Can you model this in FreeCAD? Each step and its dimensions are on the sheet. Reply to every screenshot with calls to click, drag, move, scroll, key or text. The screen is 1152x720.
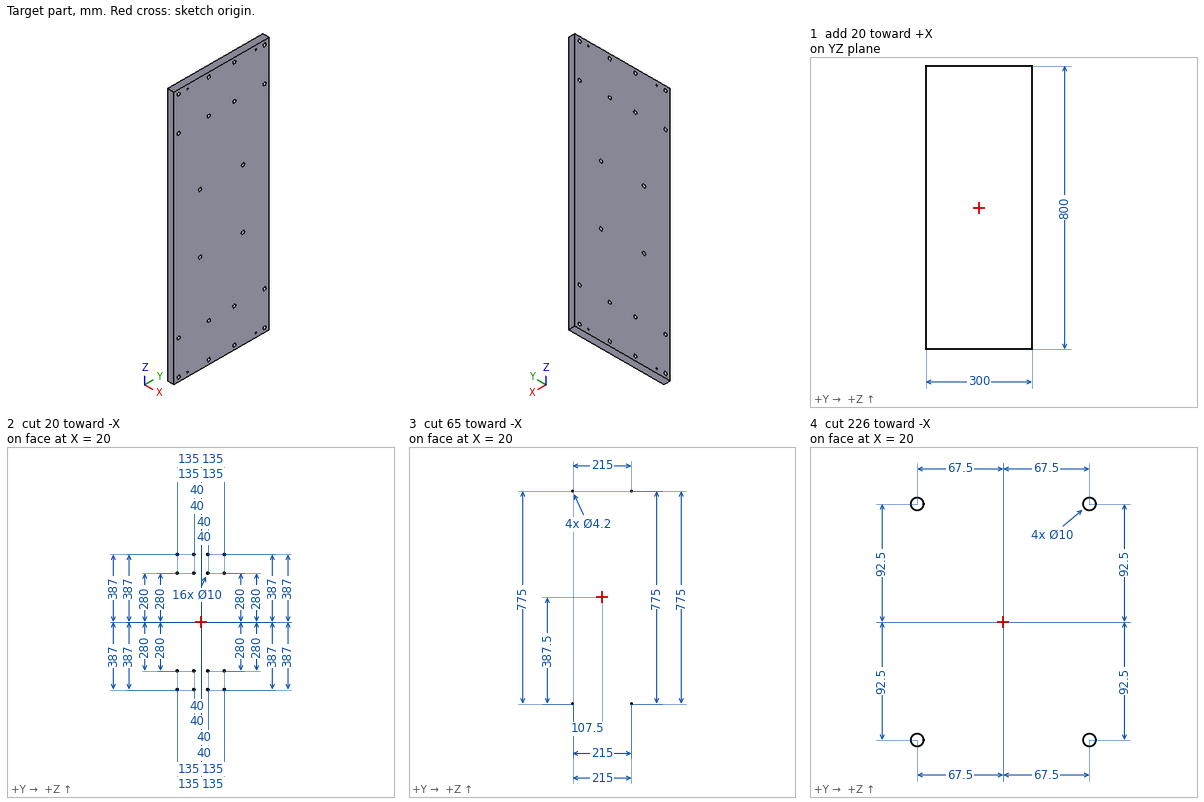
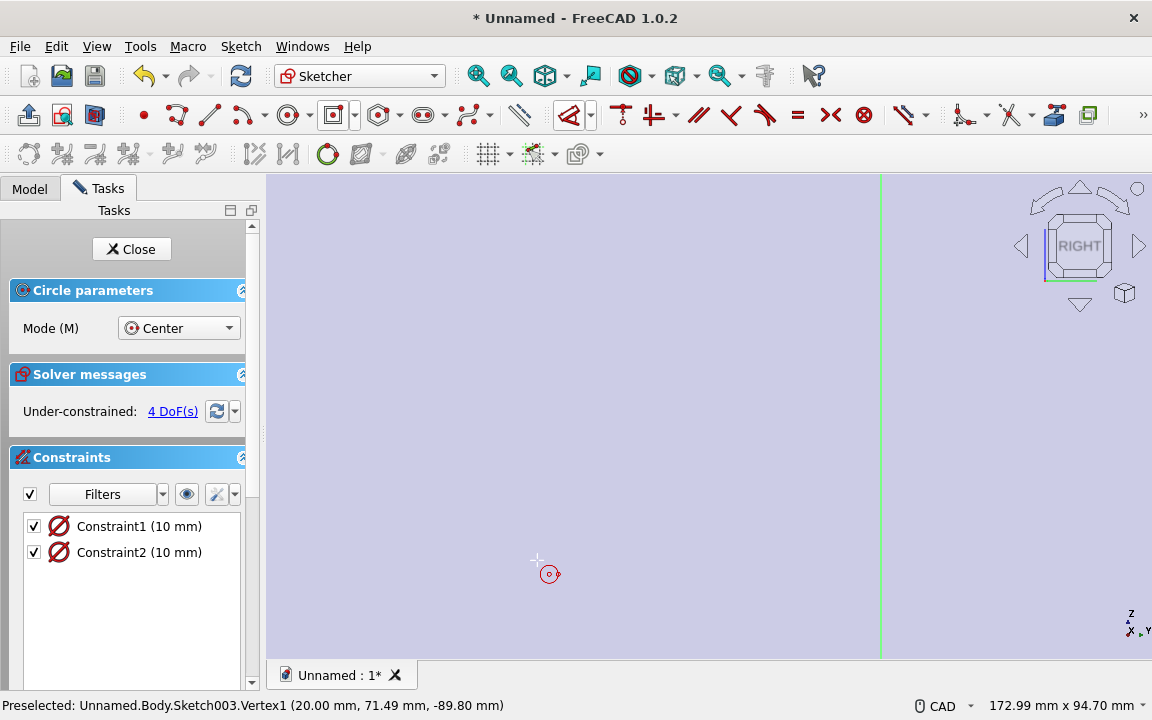
click(535, 558)
move(553, 540)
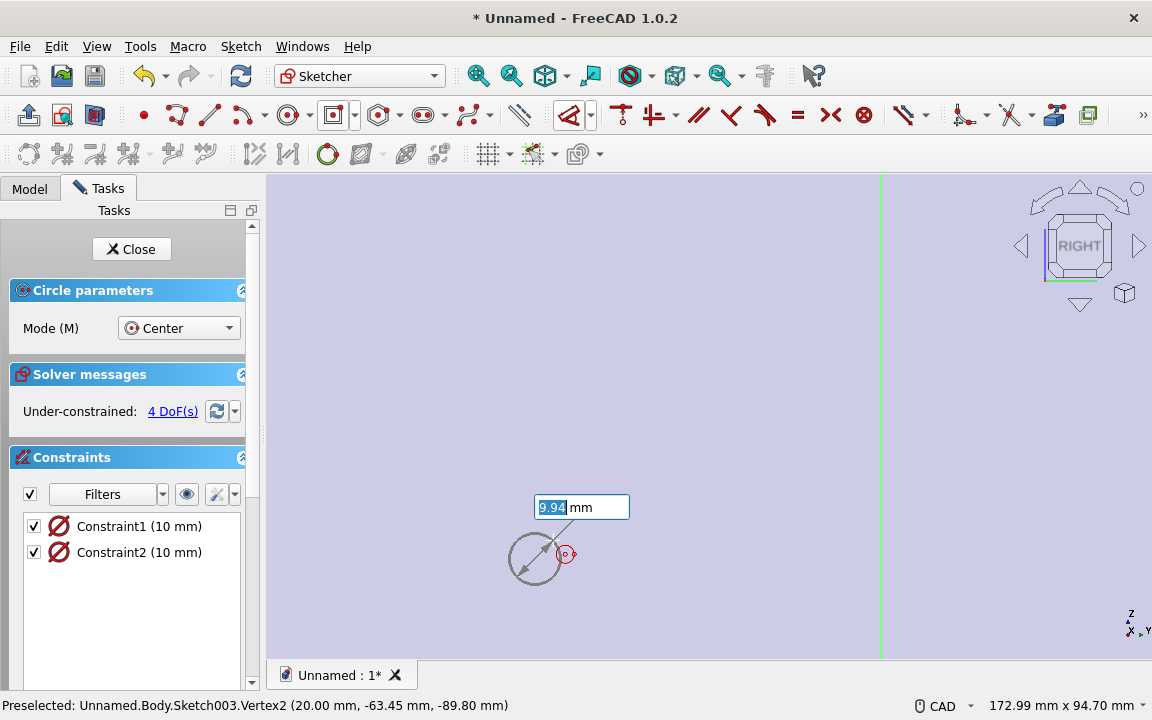
text(10)
key(Return)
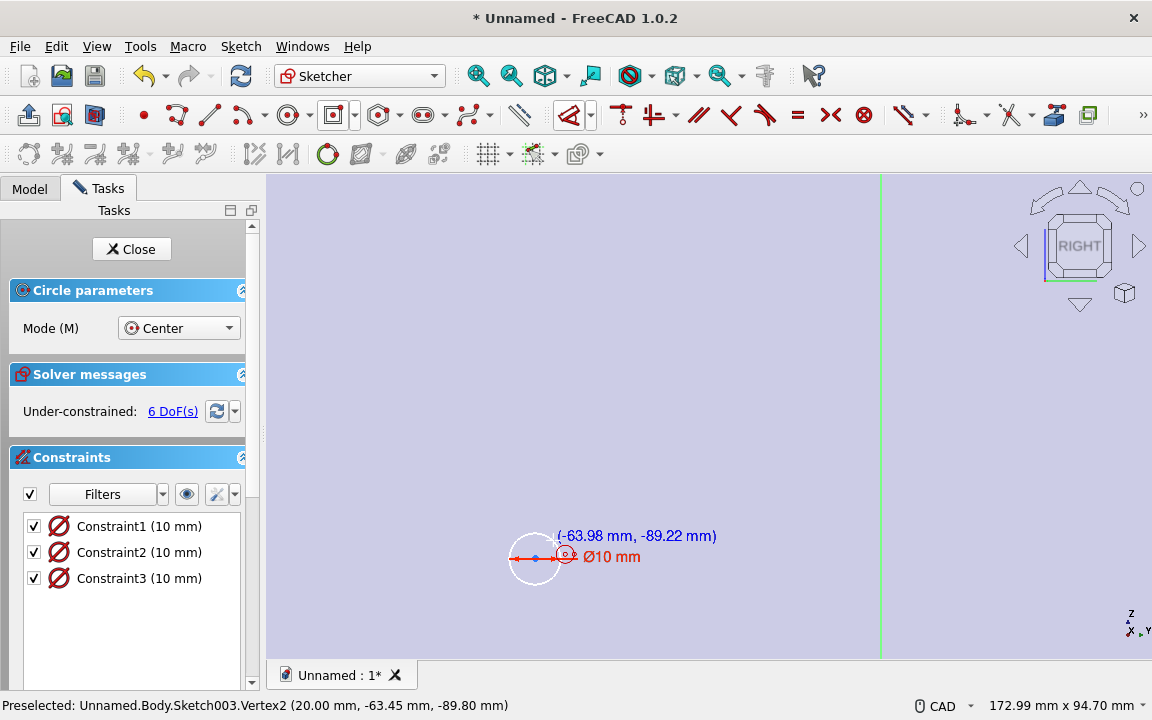
scroll(537, 560, down, 6)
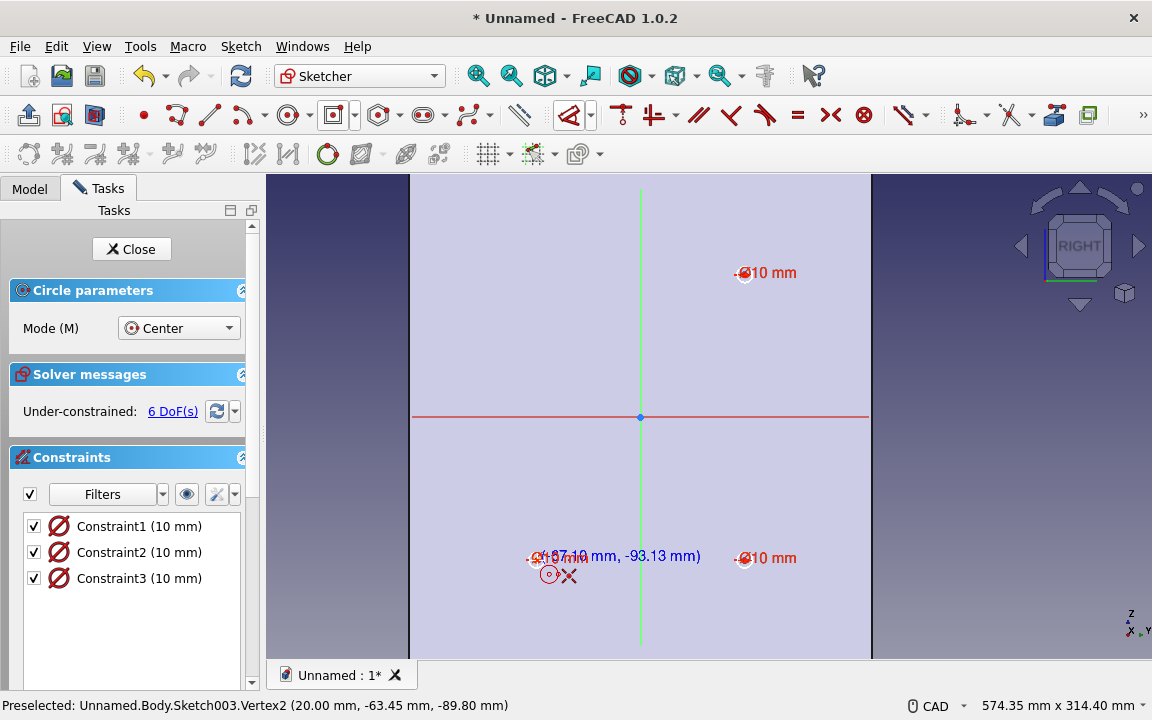
scroll(537, 275, up, 6)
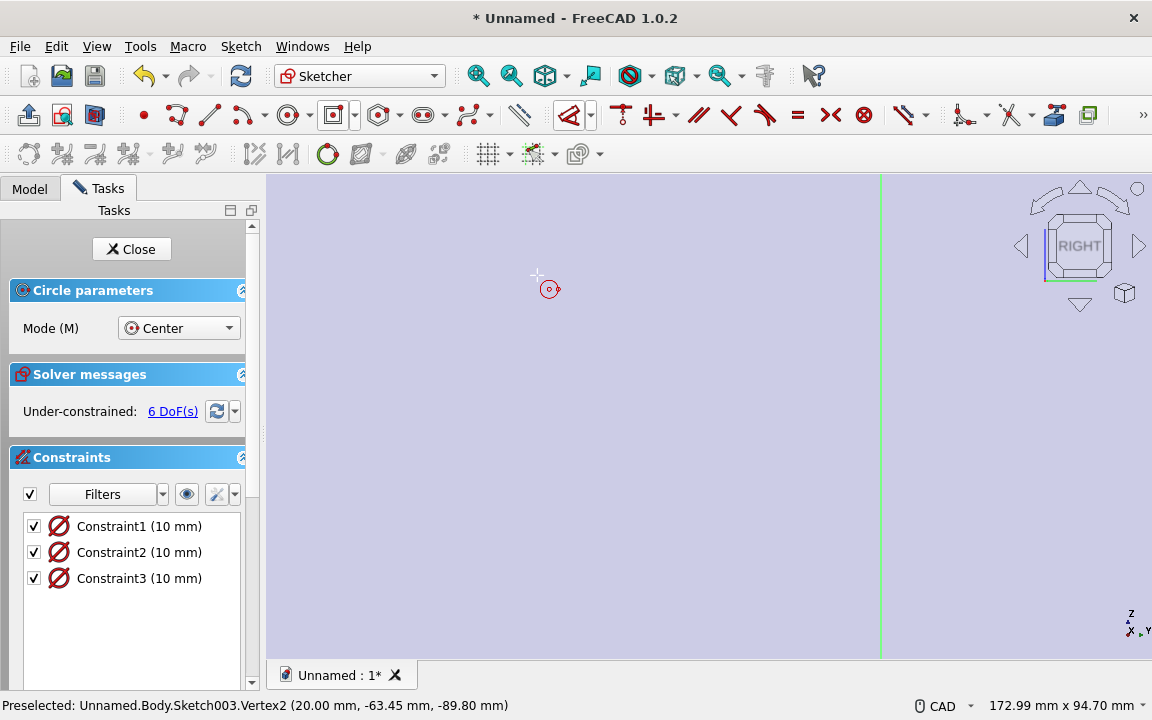
click(535, 273)
move(553, 255)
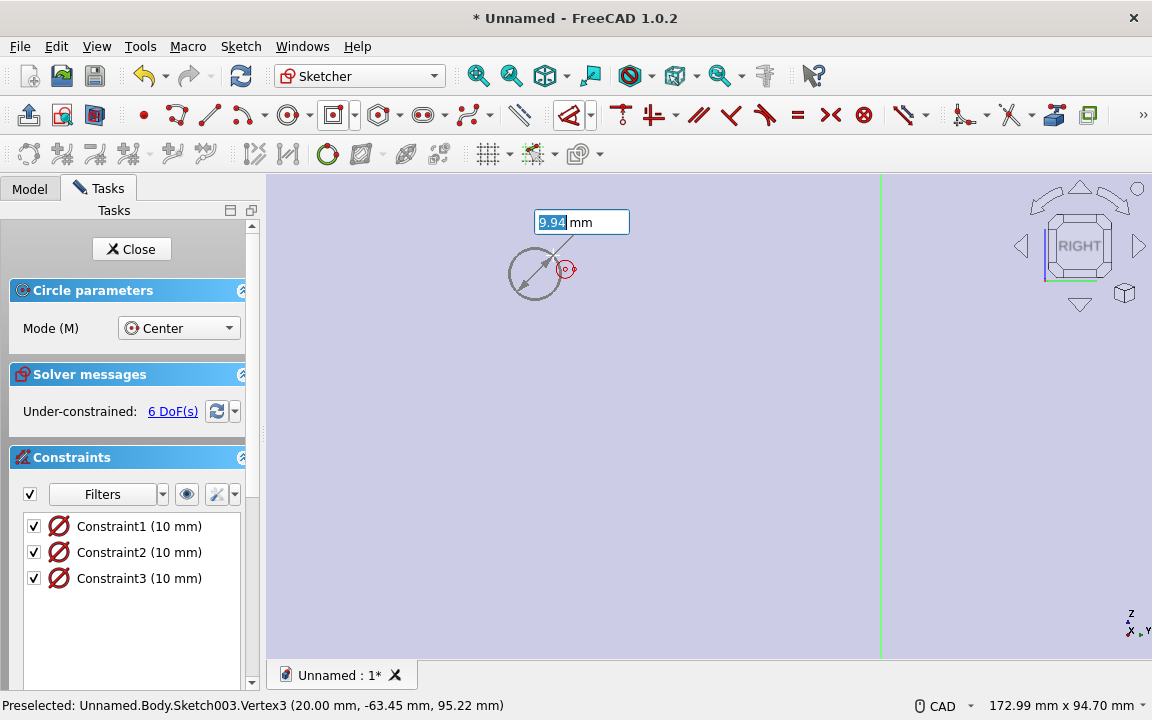
text(10)
key(Return)
key(Escape)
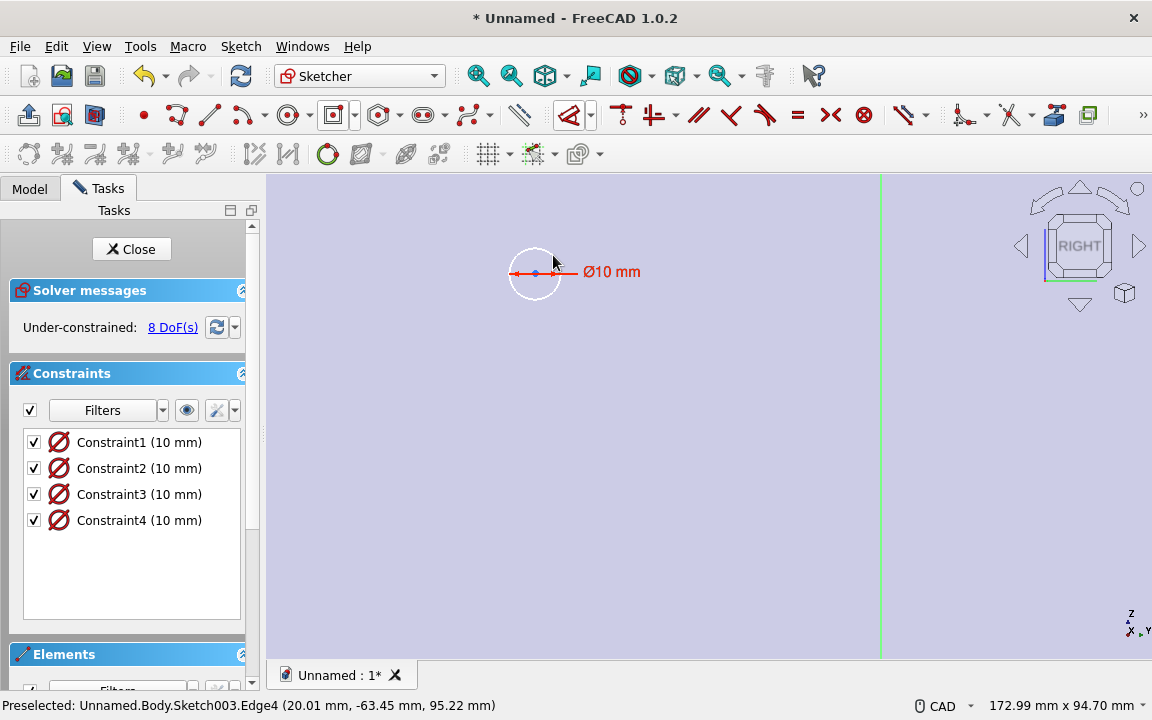
scroll(537, 274, down, 6)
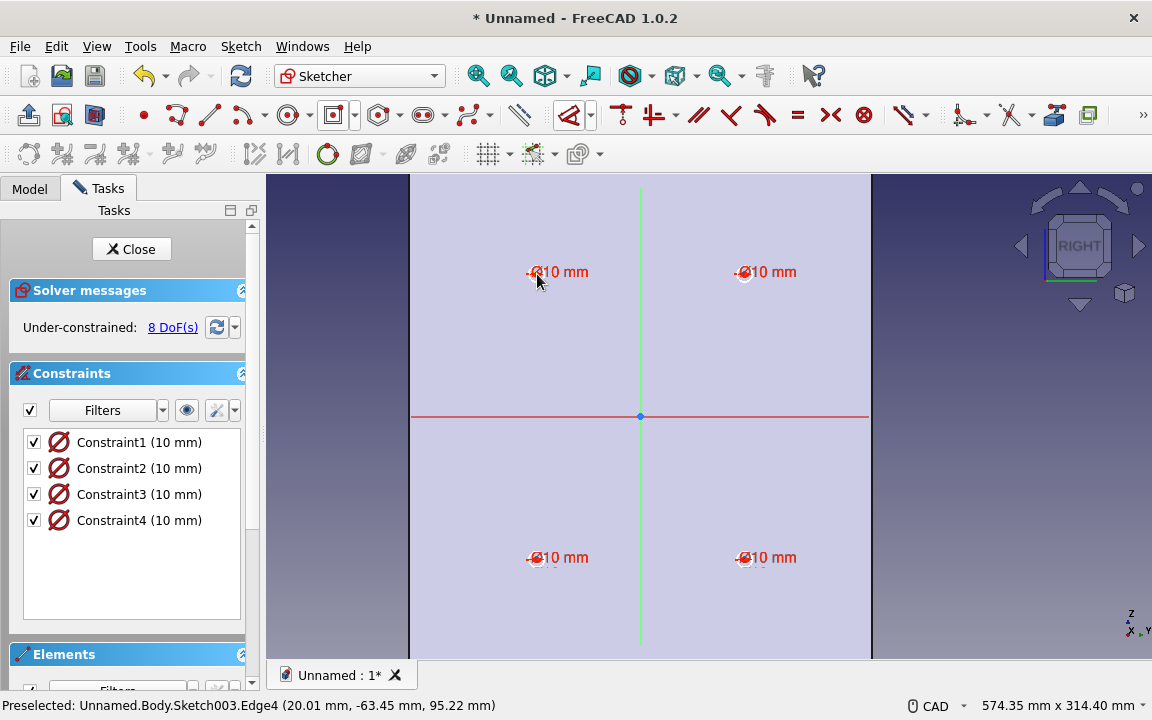
click(745, 274)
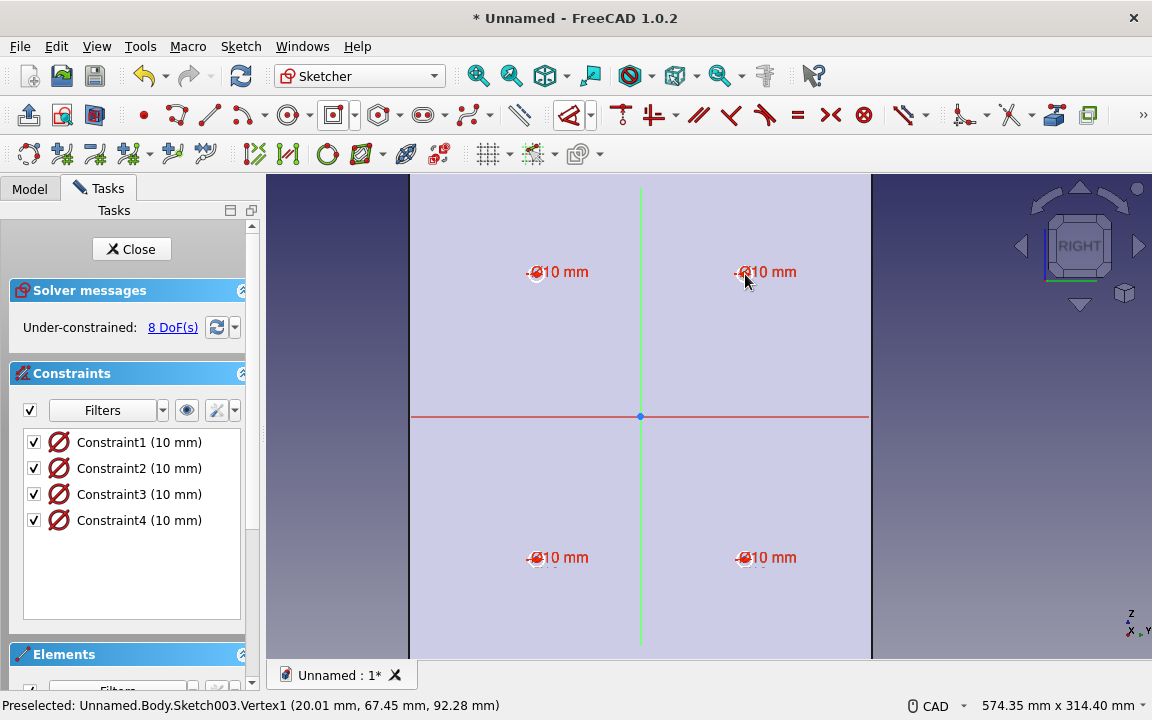
click(590, 116)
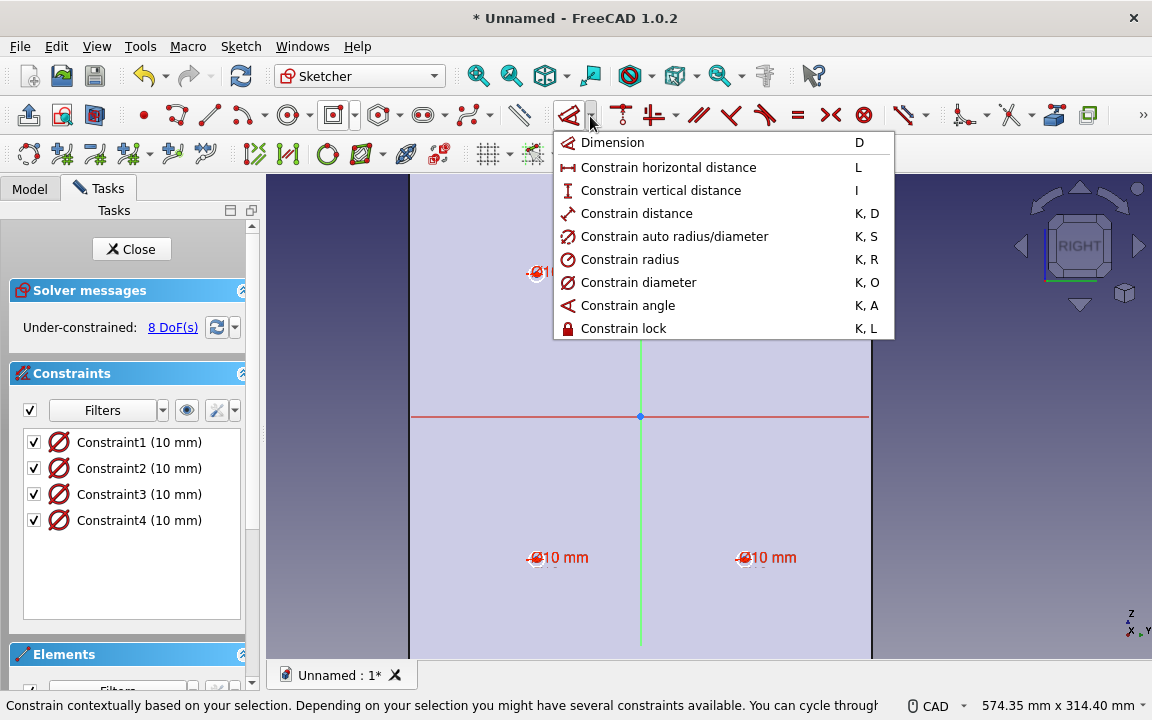
click(724, 168)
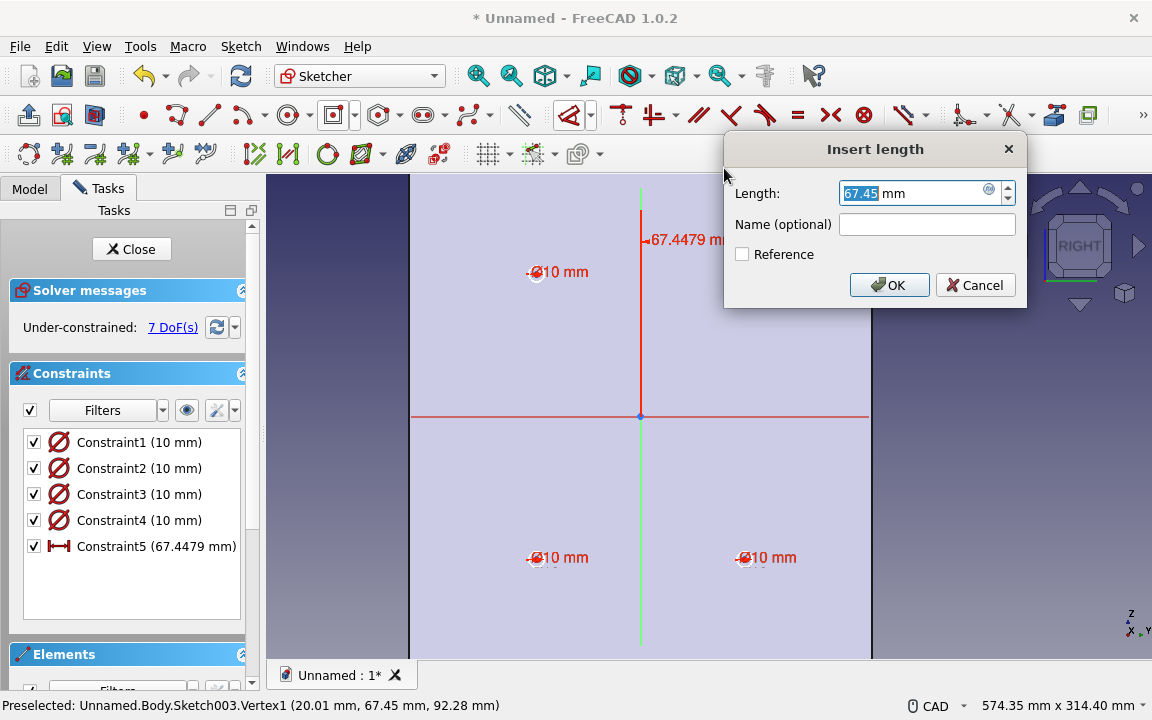
text(67.5)
key(Return)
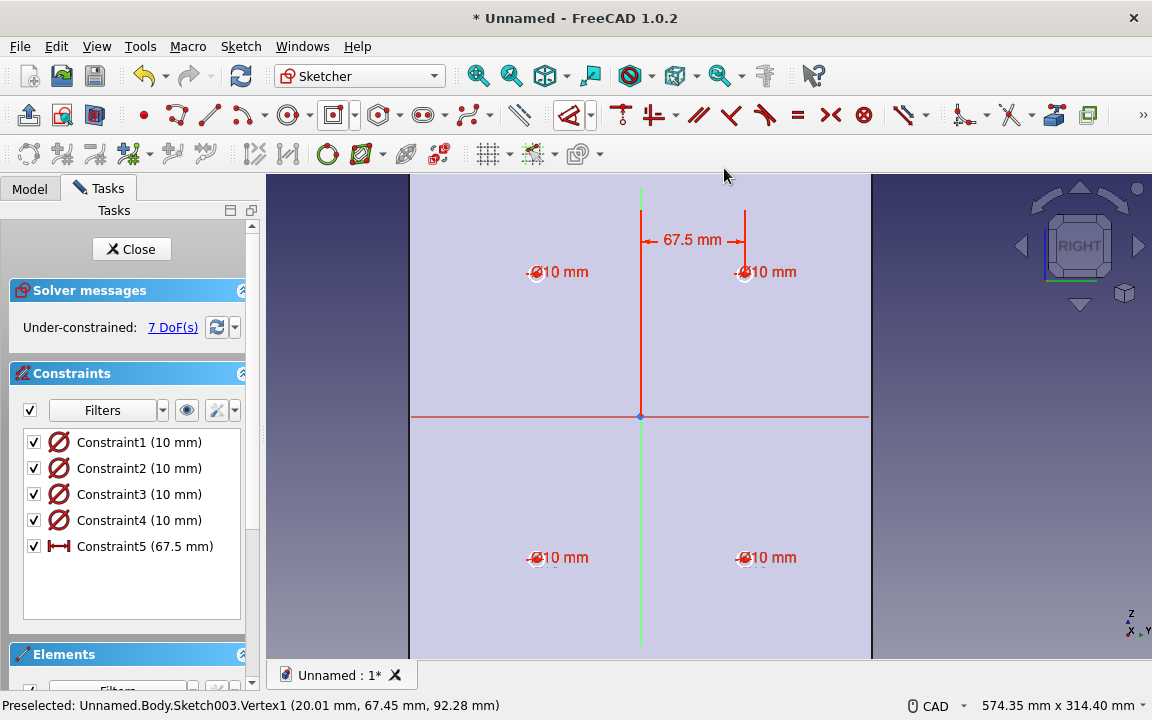
click(745, 274)